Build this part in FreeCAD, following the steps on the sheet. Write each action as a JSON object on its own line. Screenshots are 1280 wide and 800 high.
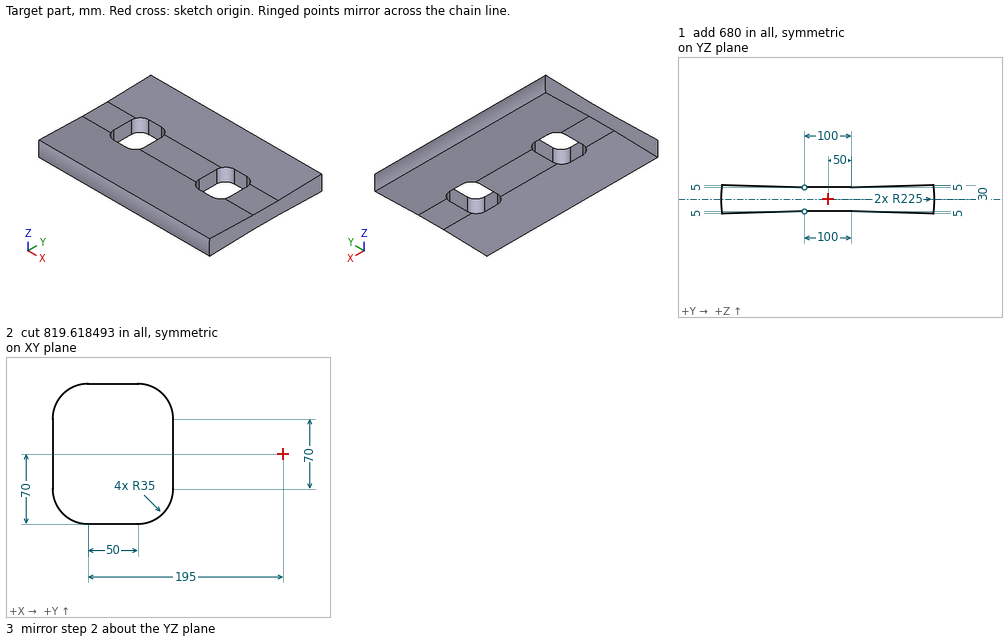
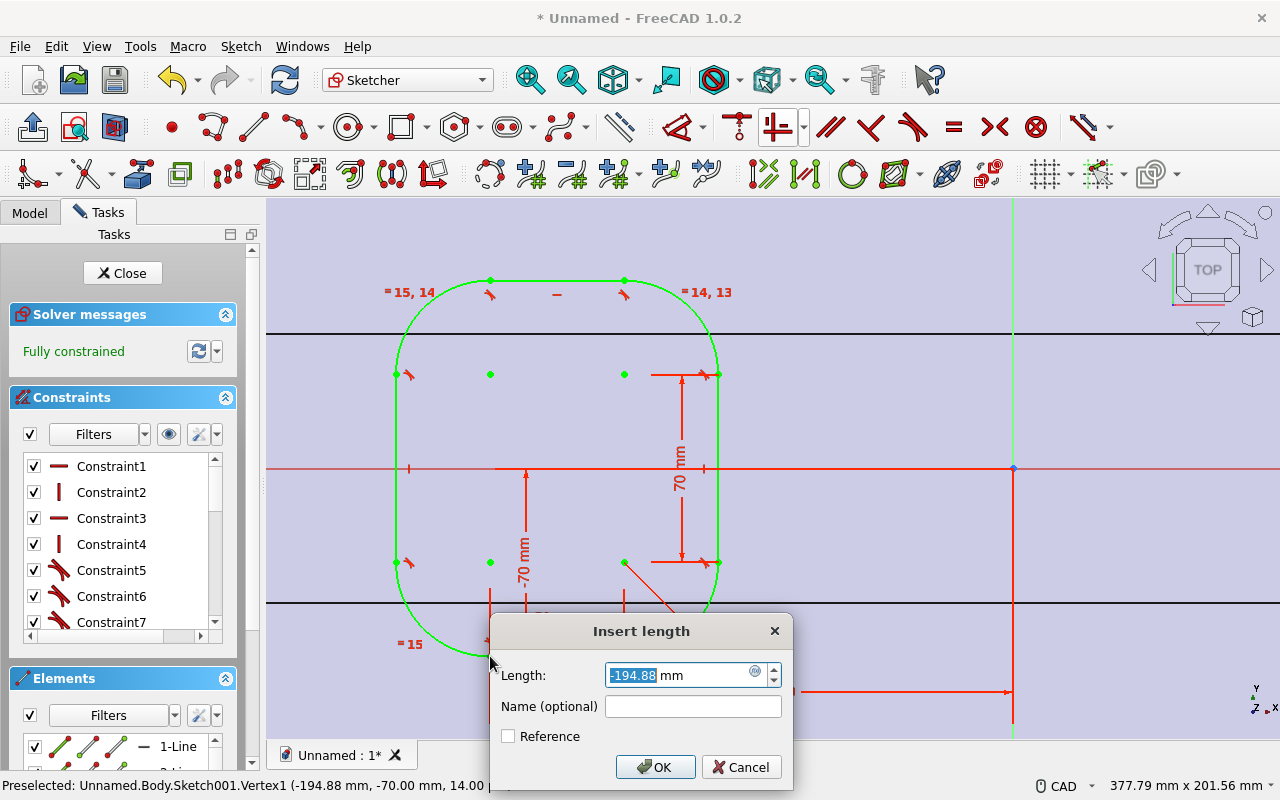
{"action": "type", "text": "-195"}
{"action": "key", "text": "Return"}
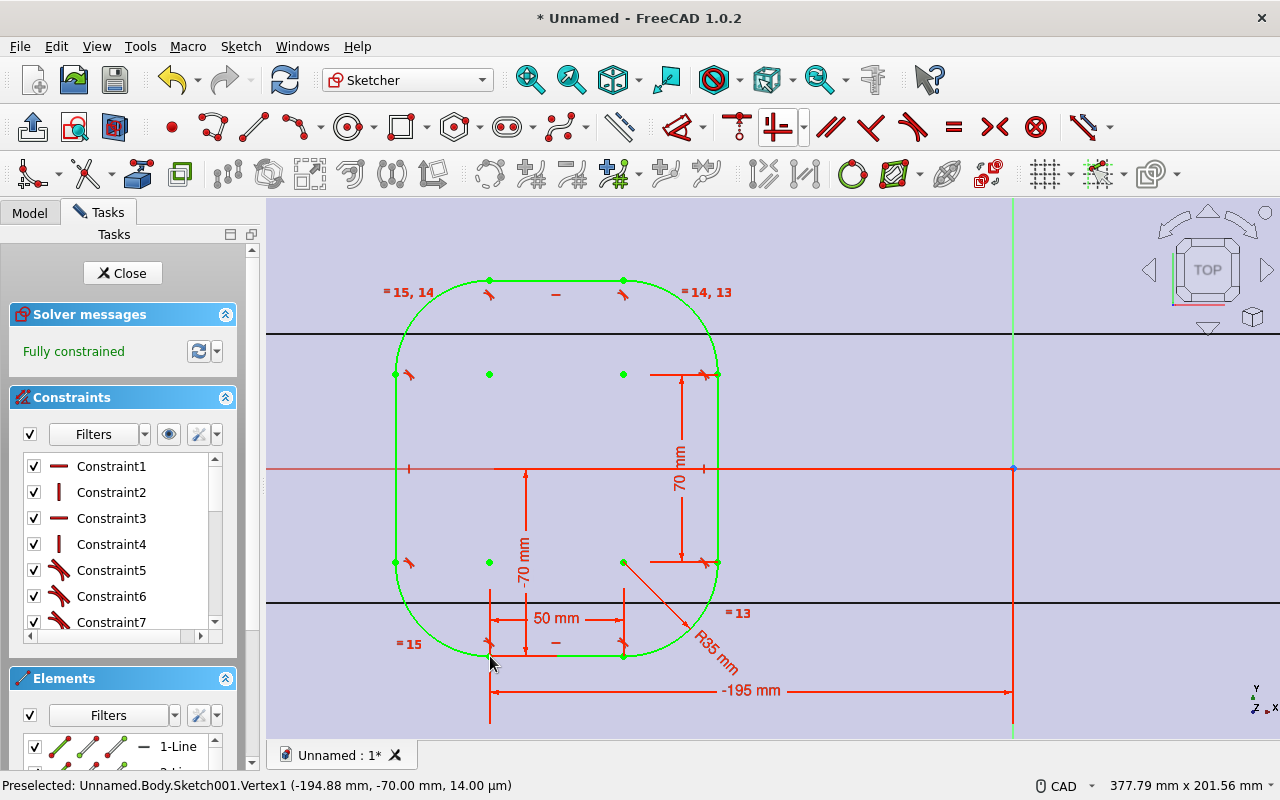
{"action": "left_click", "coordinate": [123, 273]}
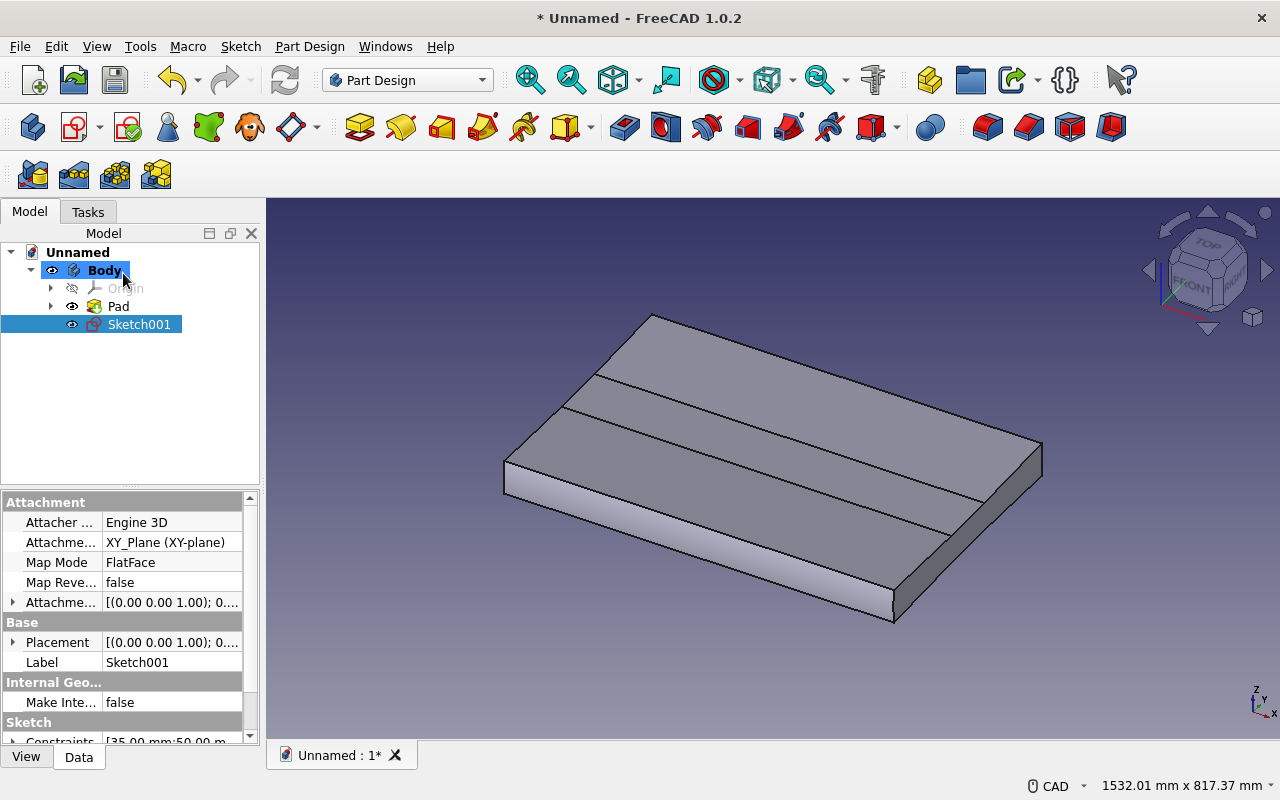
{"action": "left_click", "coordinate": [625, 128]}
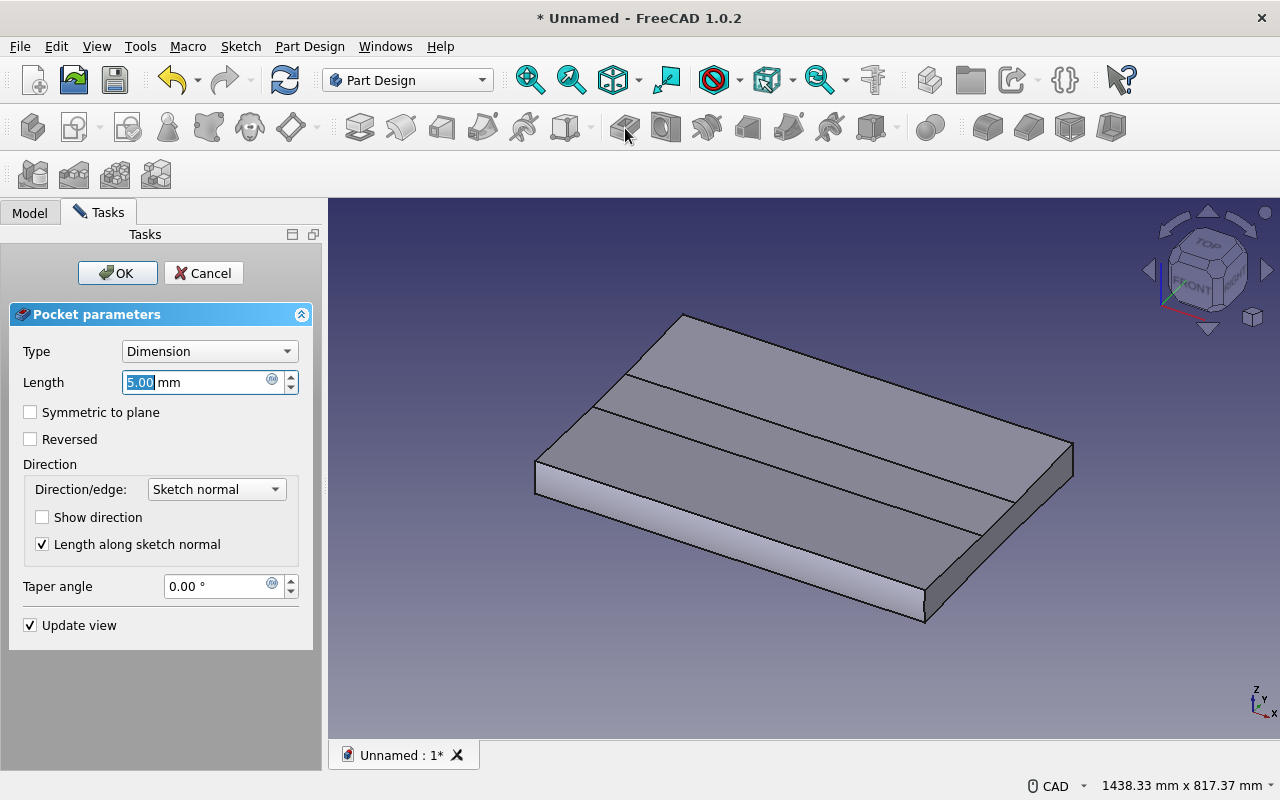
{"action": "type", "text": "819.618493"}
{"action": "key", "text": "Tab"}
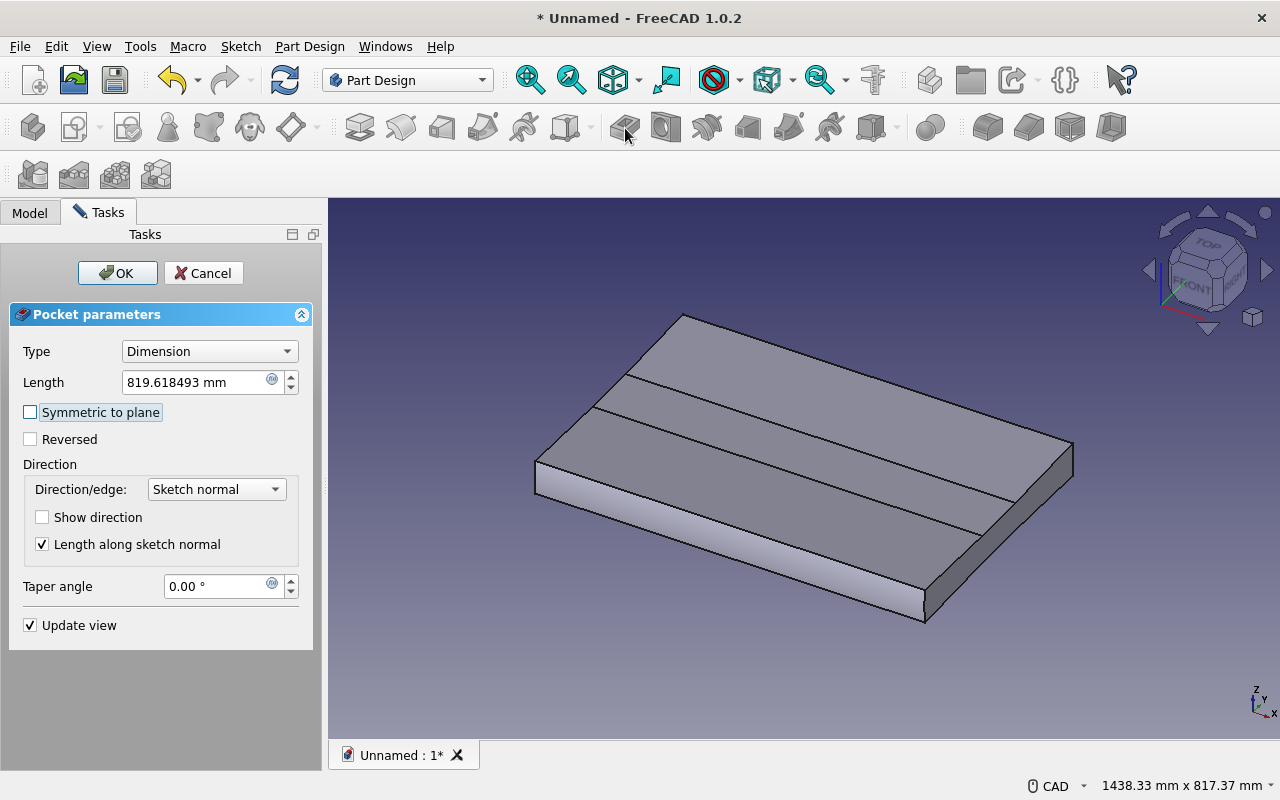
{"action": "left_click", "coordinate": [31, 412]}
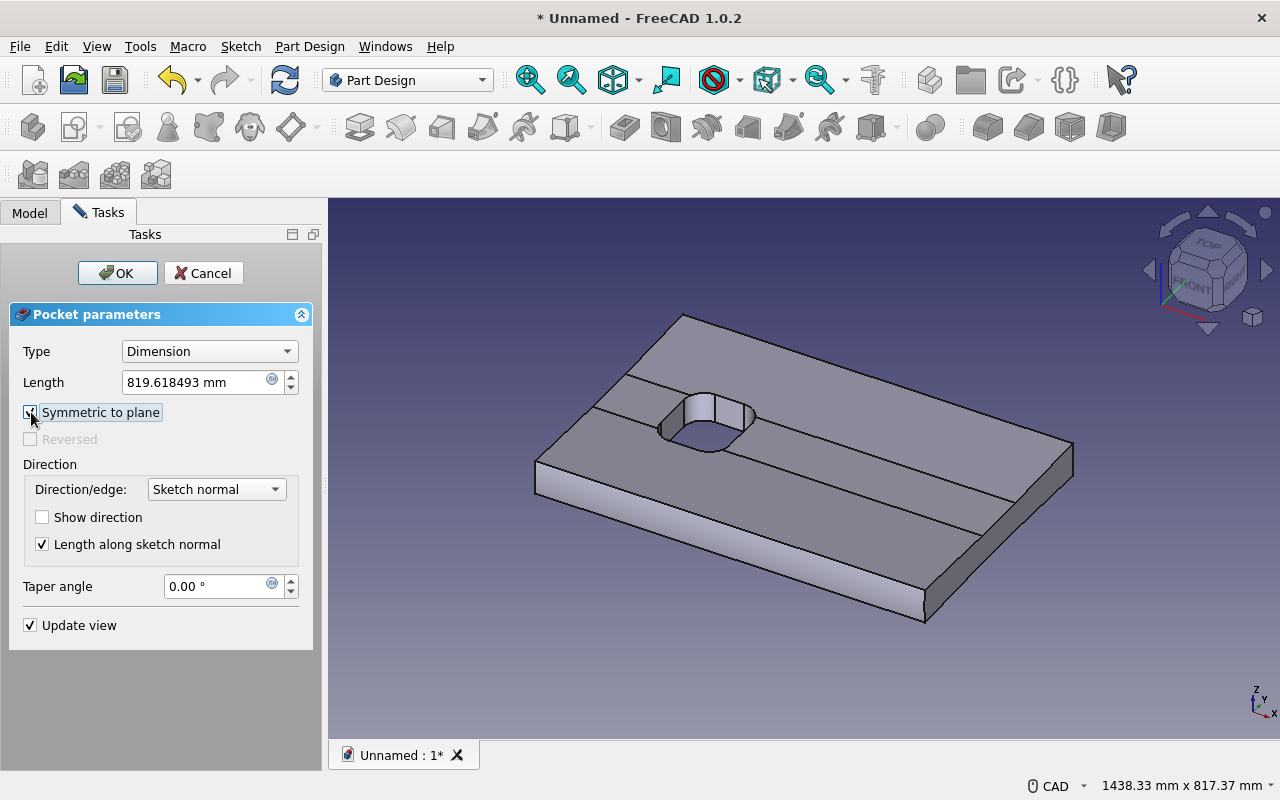
{"action": "left_click", "coordinate": [118, 273]}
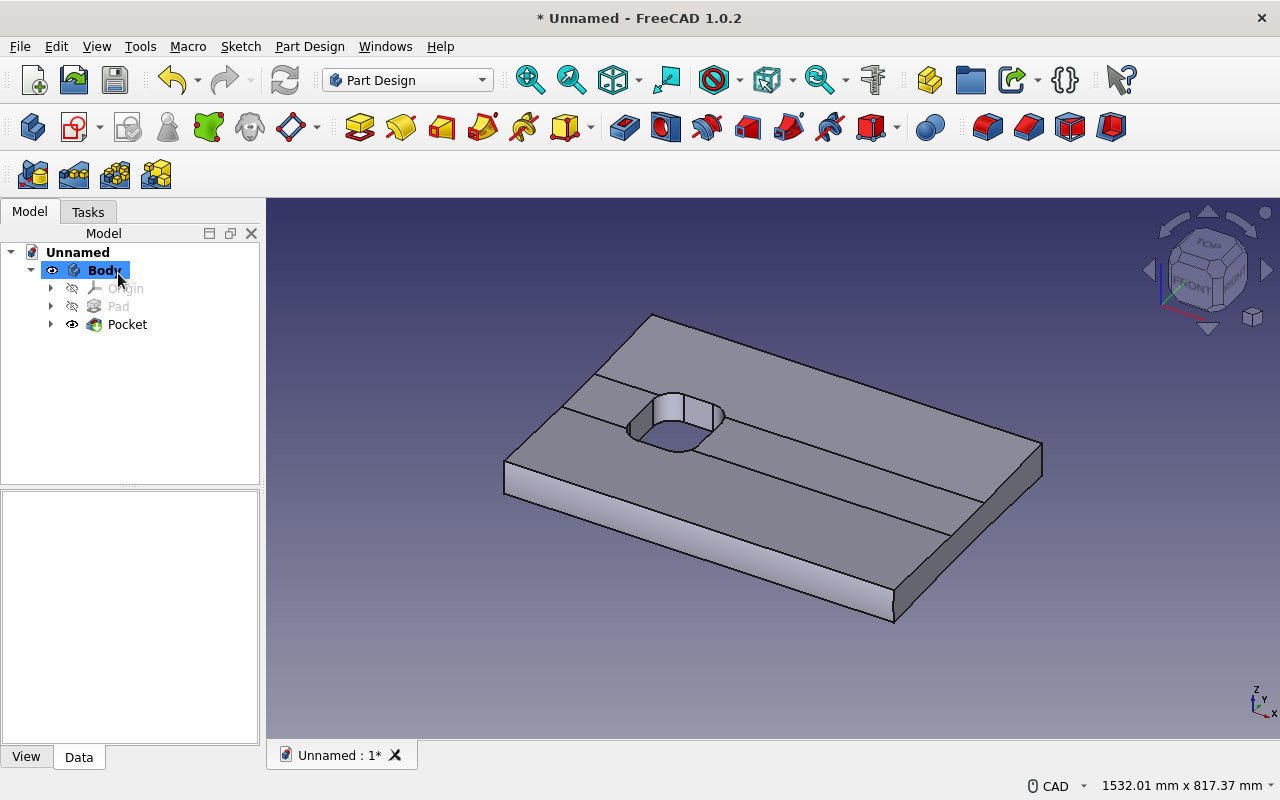
{"action": "left_click", "coordinate": [117, 324]}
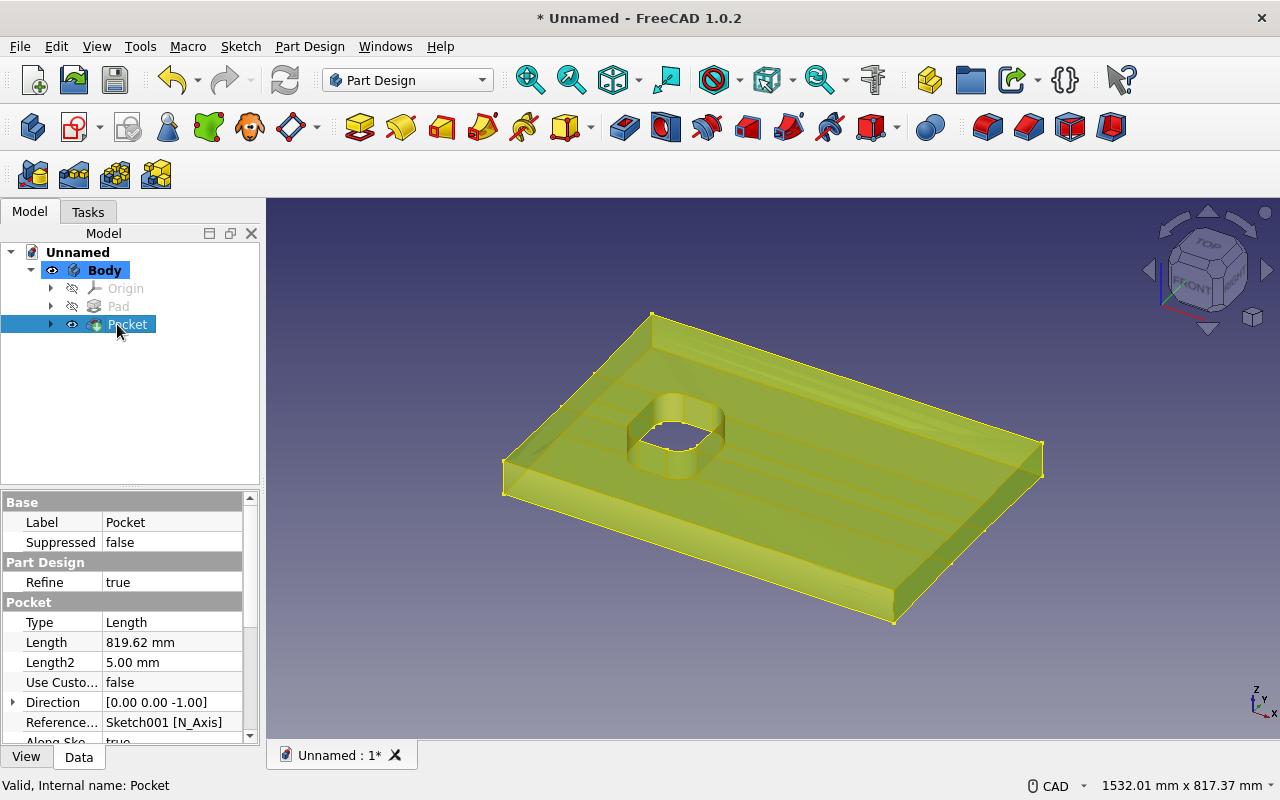
{"action": "left_click", "coordinate": [33, 174]}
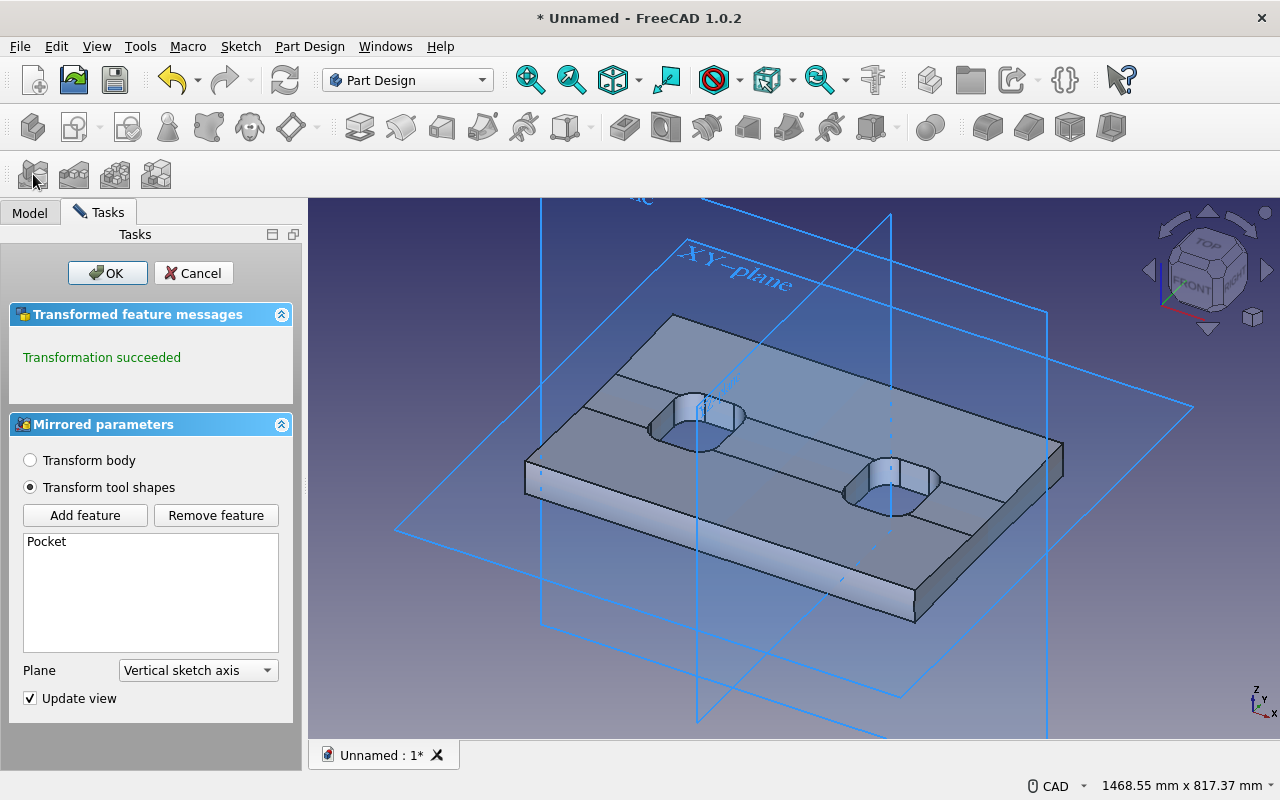
{"action": "left_click", "coordinate": [199, 670]}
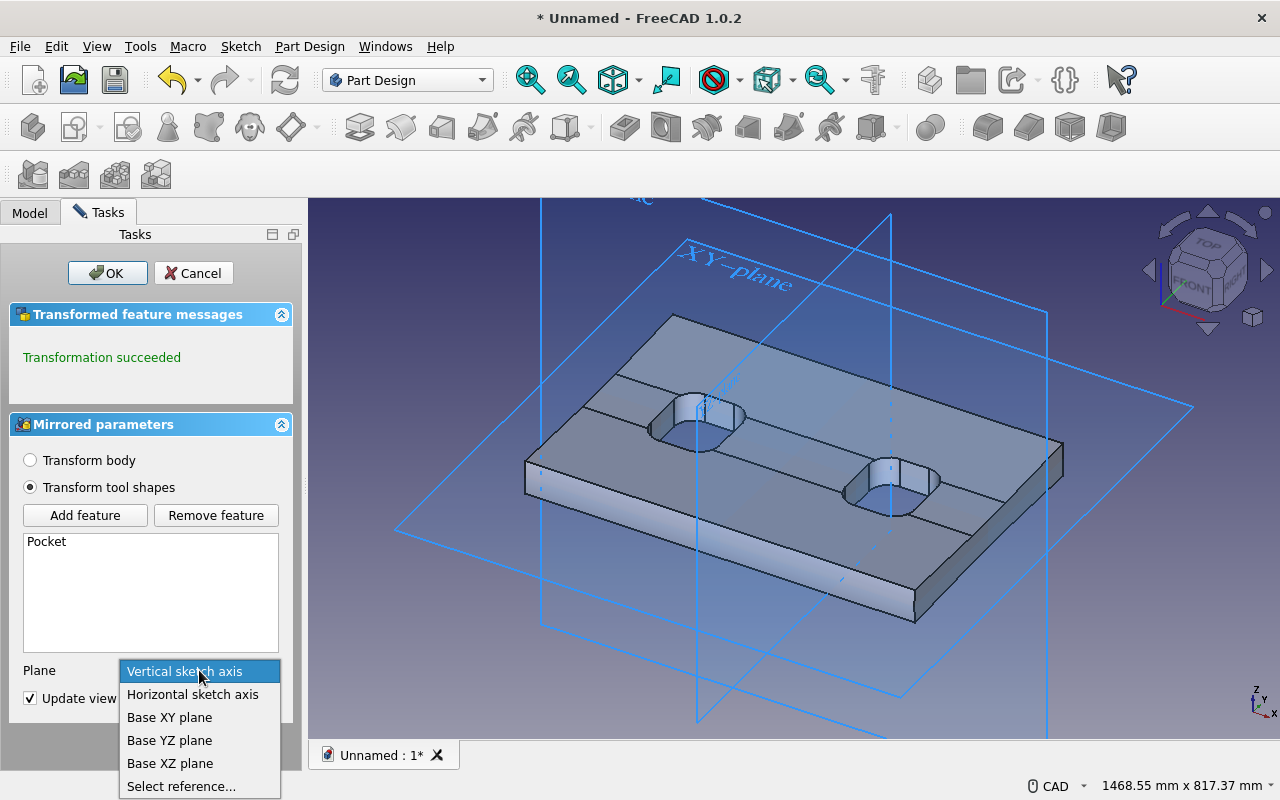
{"action": "left_click", "coordinate": [198, 740]}